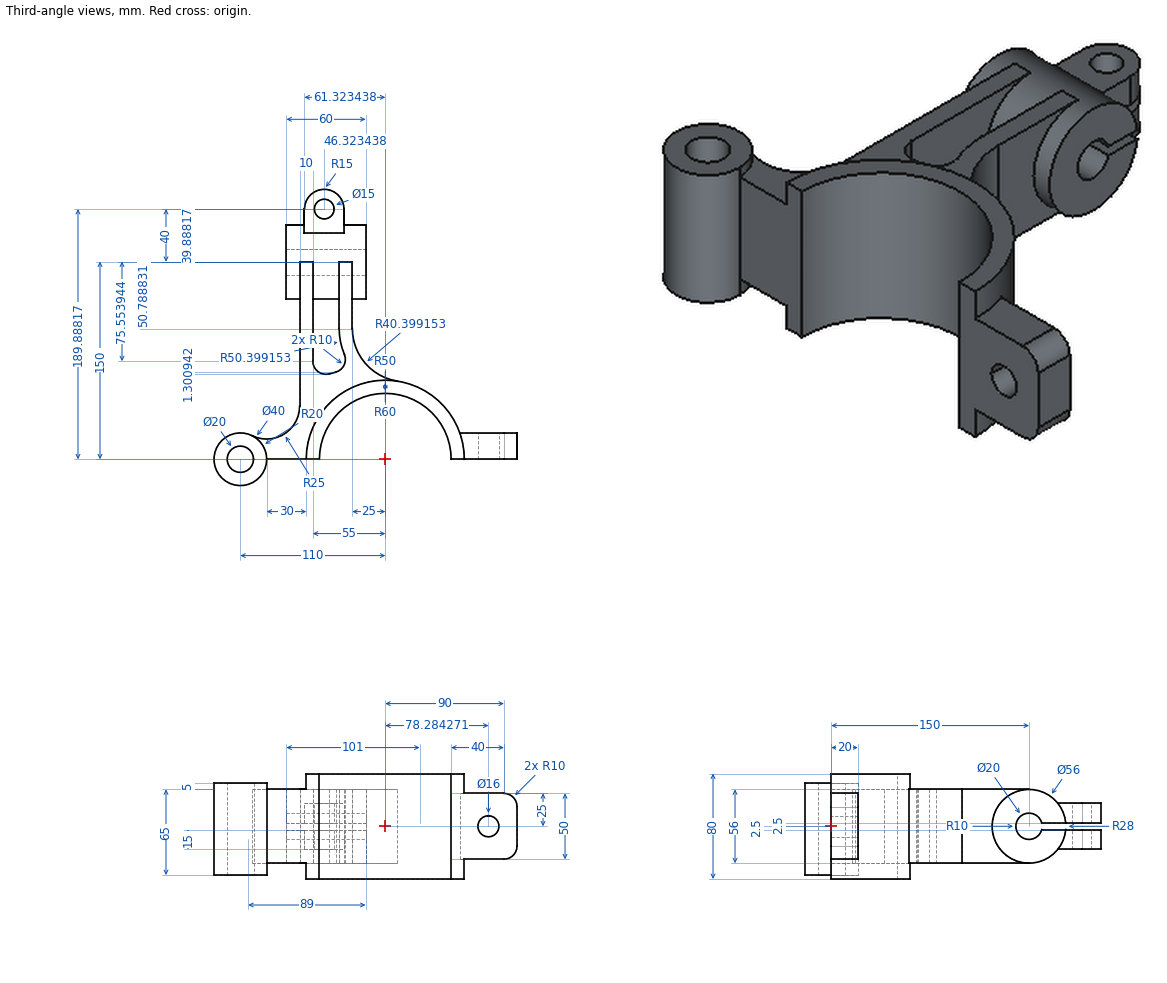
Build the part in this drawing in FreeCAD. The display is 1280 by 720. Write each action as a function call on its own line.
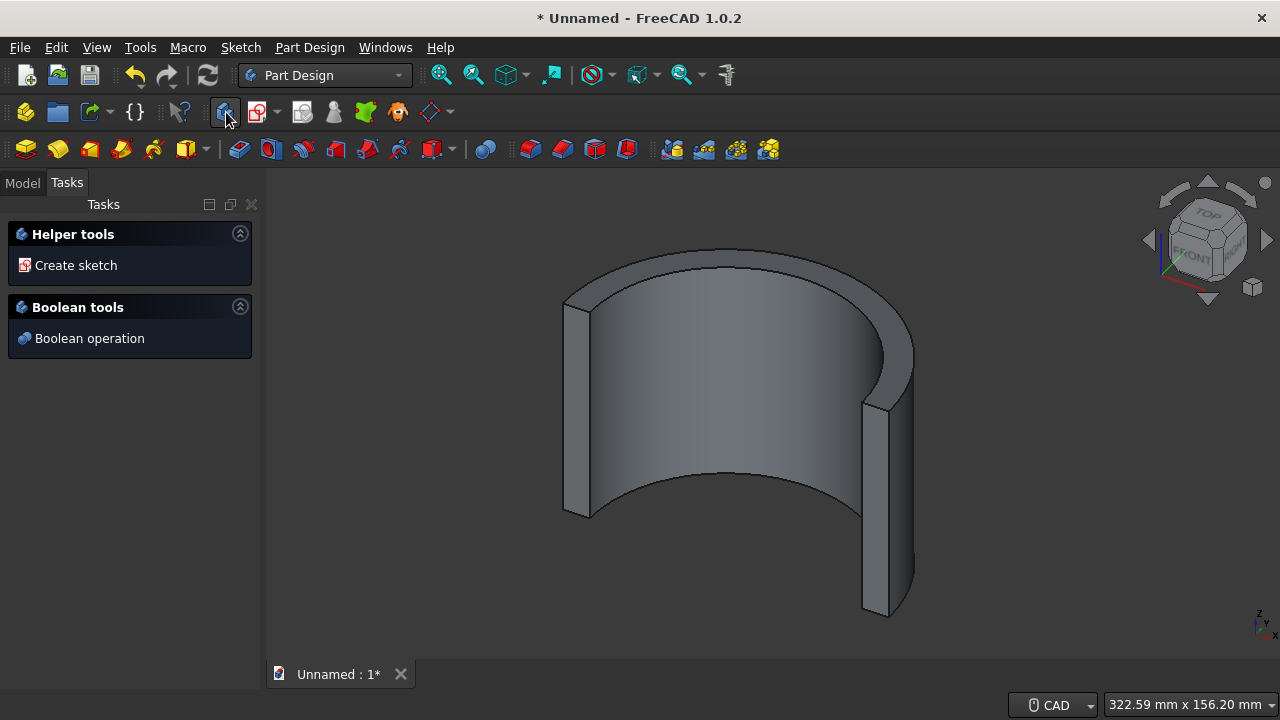
click(23, 182)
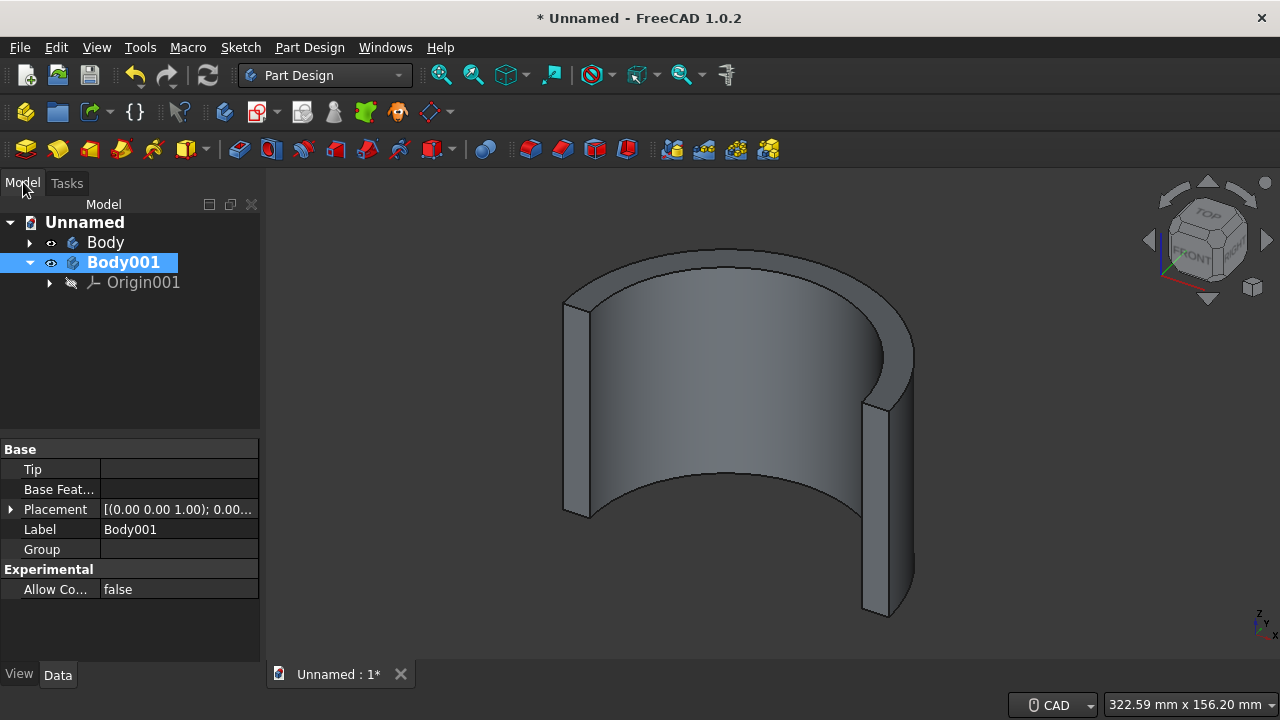
click(50, 283)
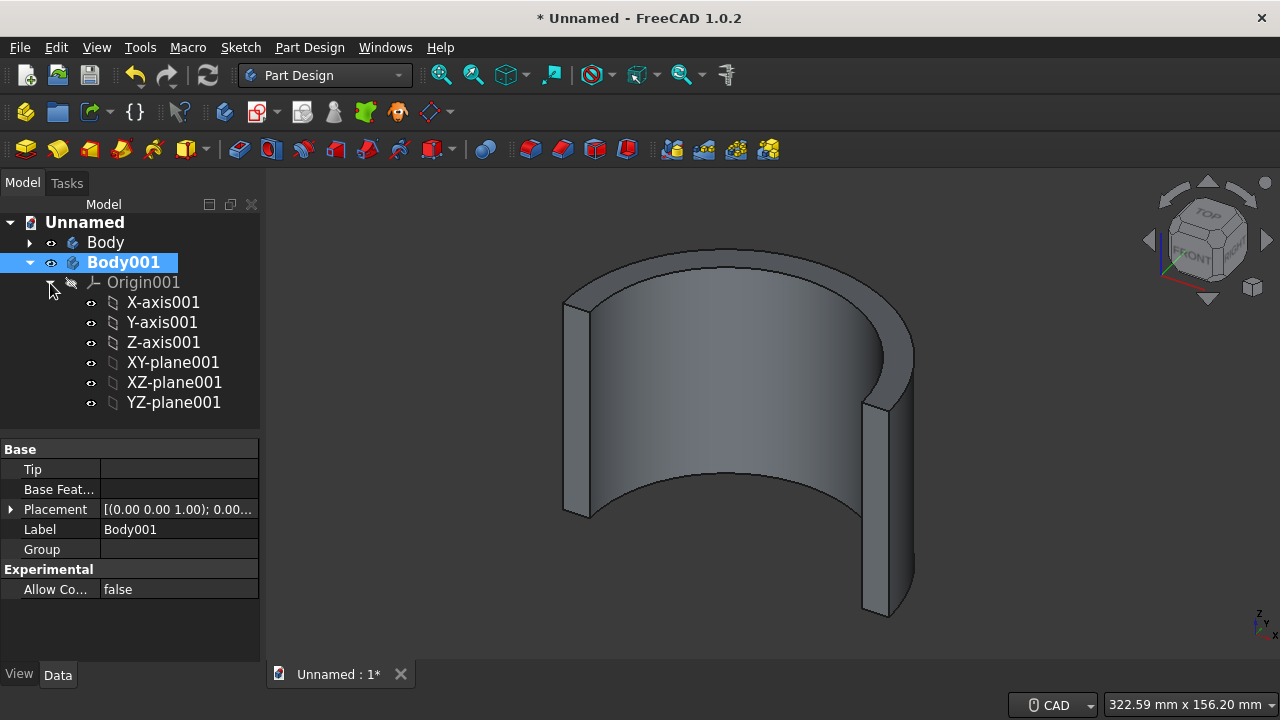
click(136, 363)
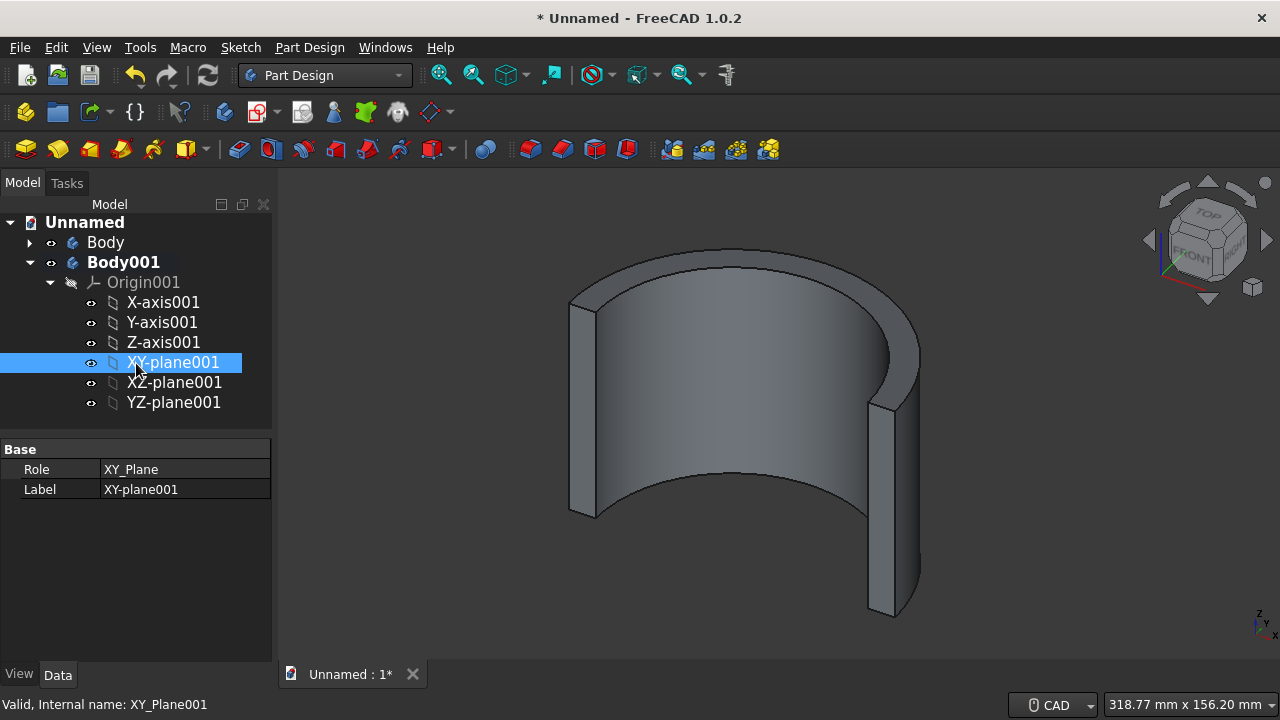
click(430, 112)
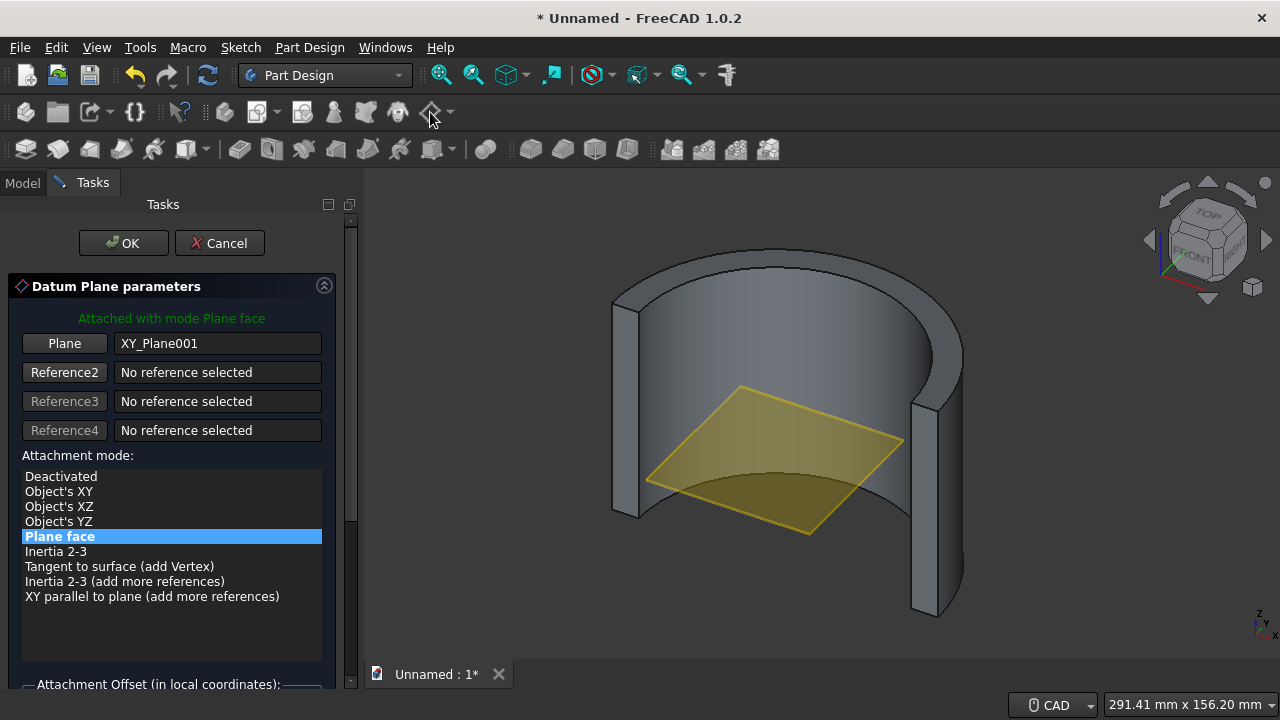
scroll(351, 451, down, 3)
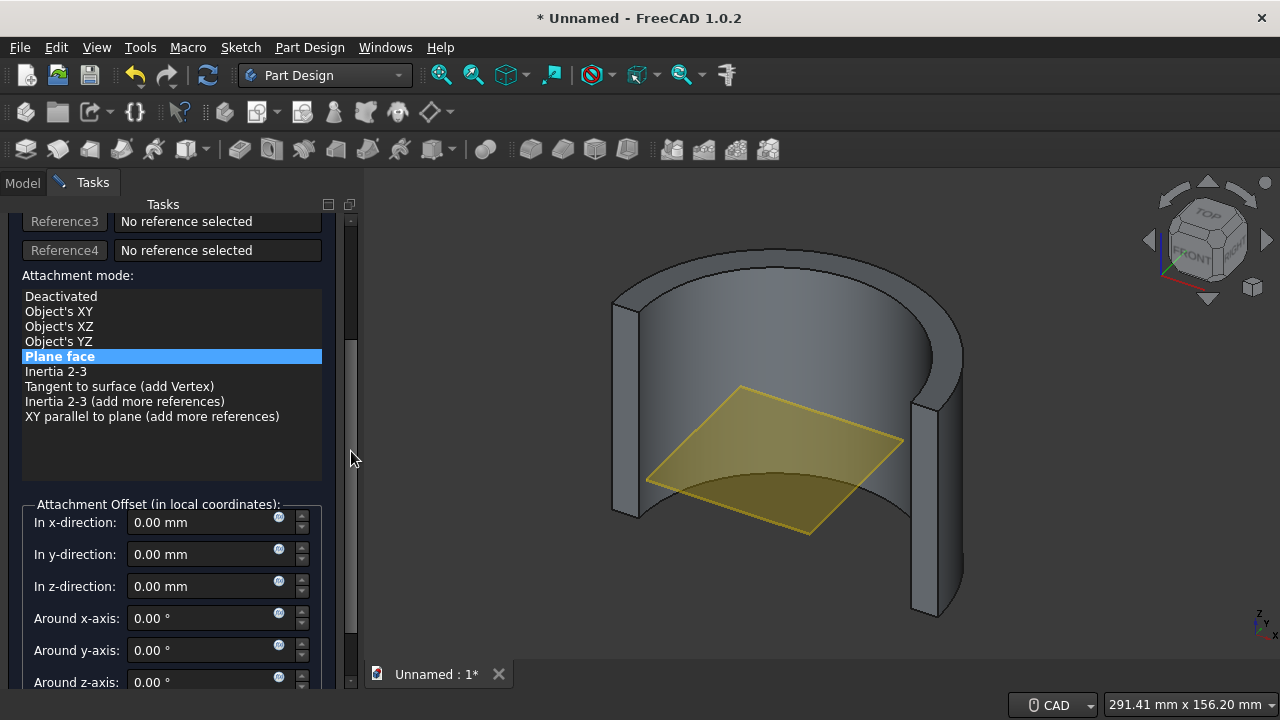
triple_click(210, 586)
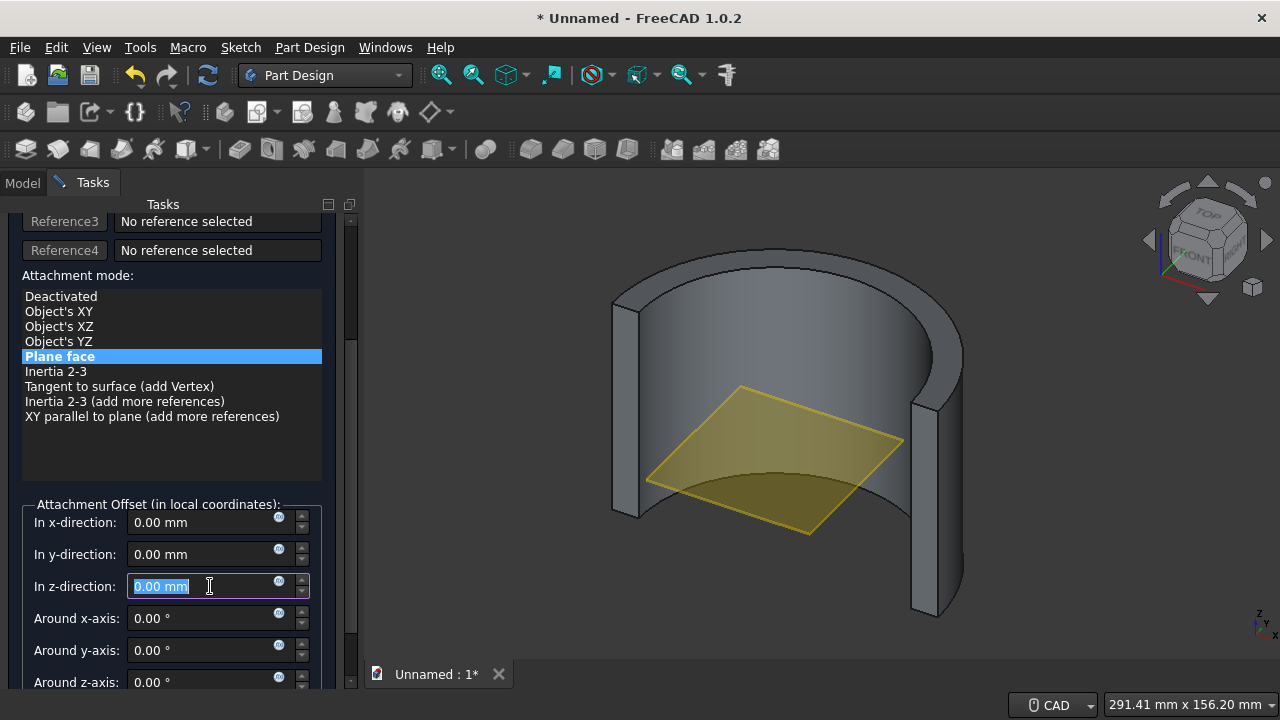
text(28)
key(Tab)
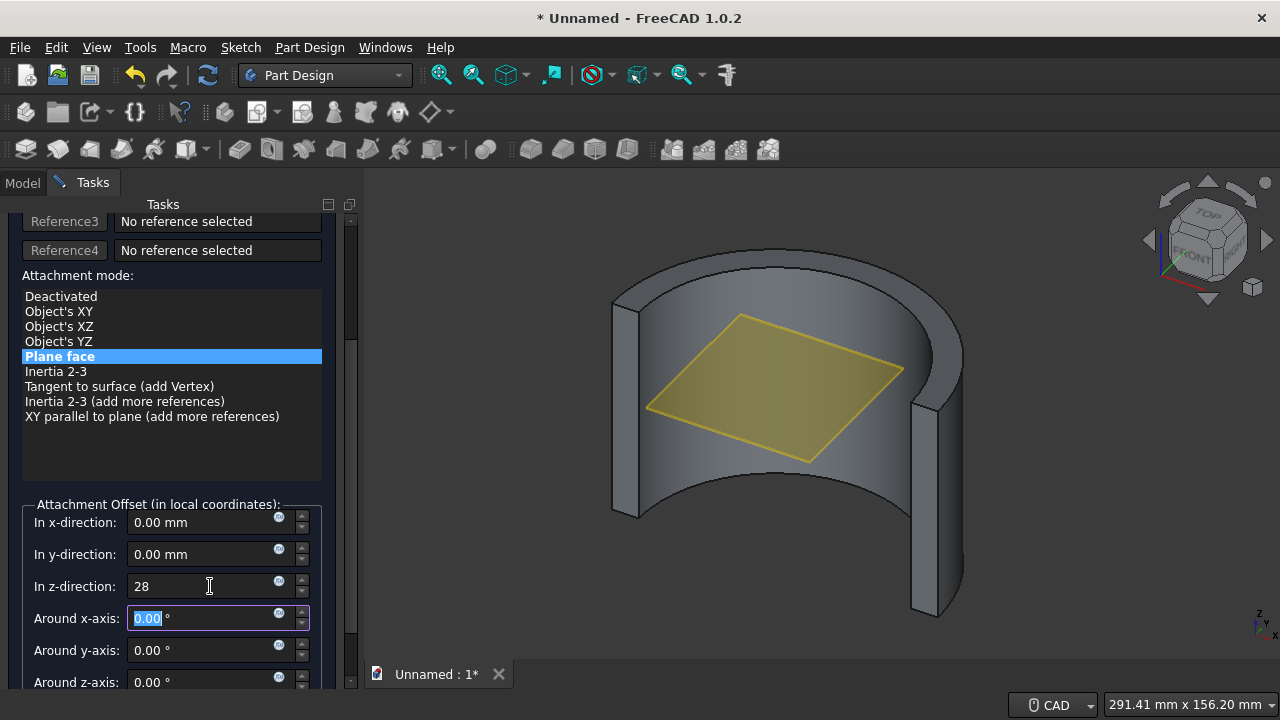
scroll(351, 451, up, 4)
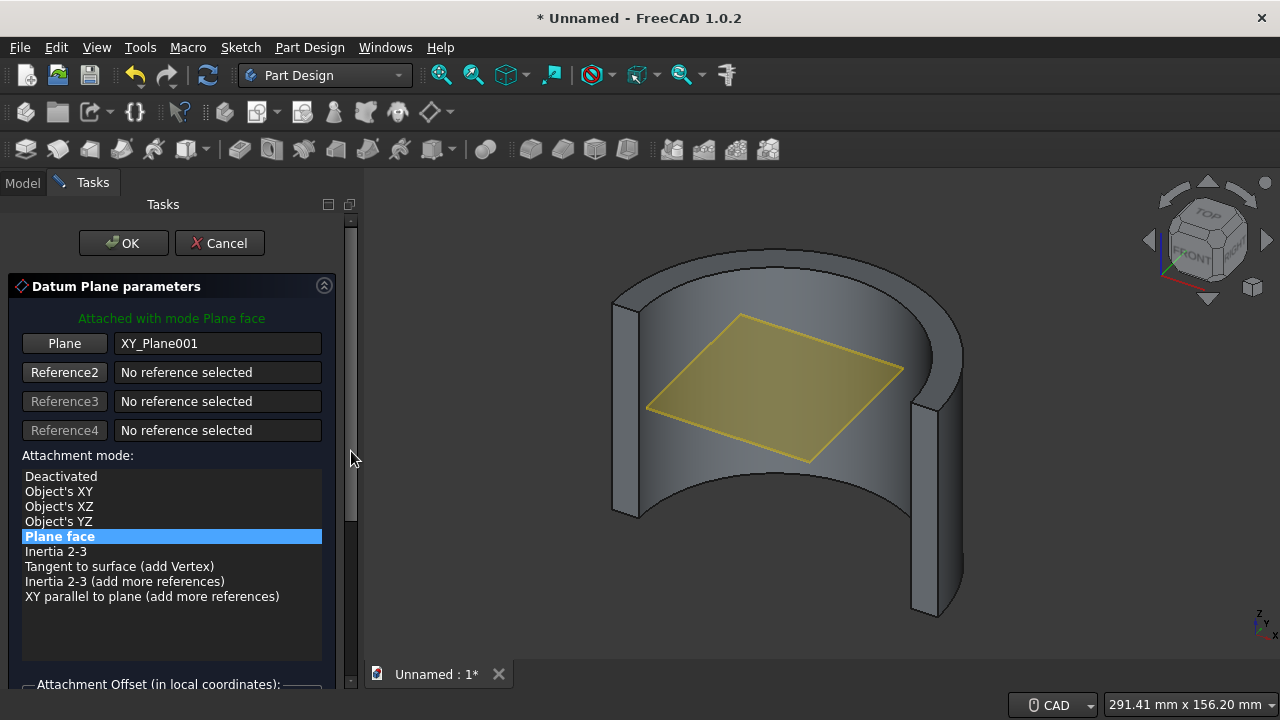
click(124, 243)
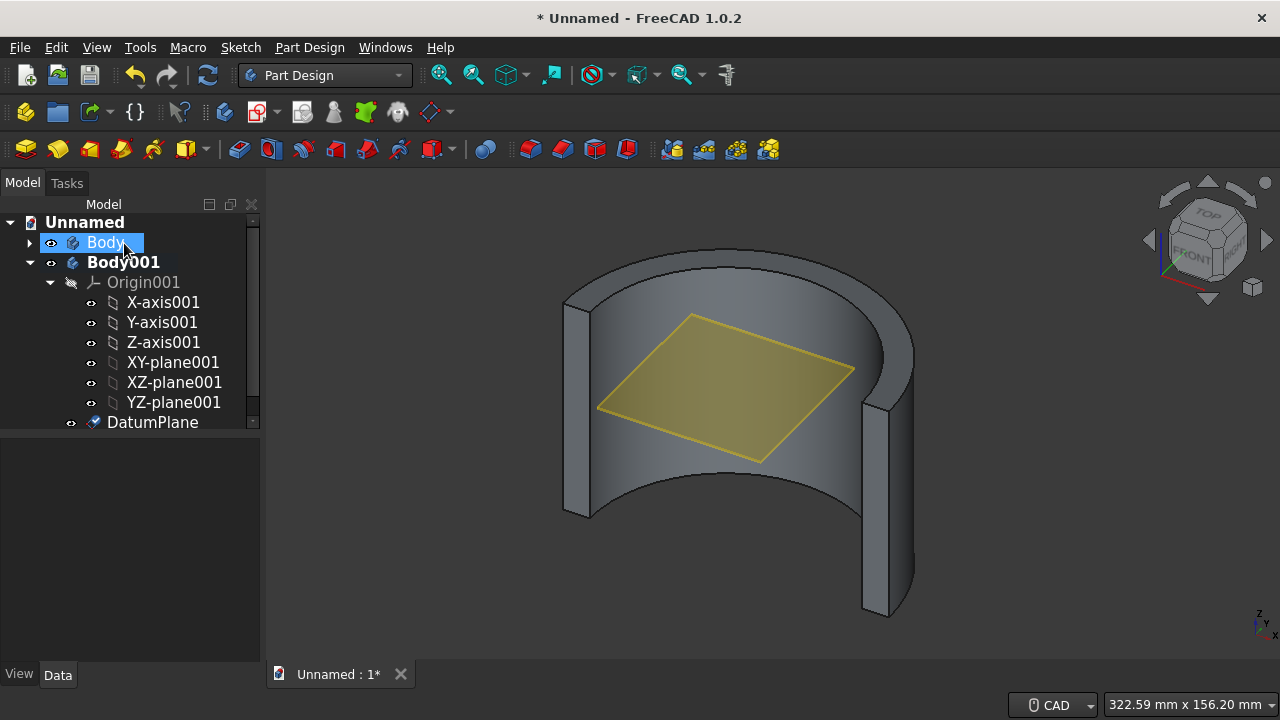
click(116, 423)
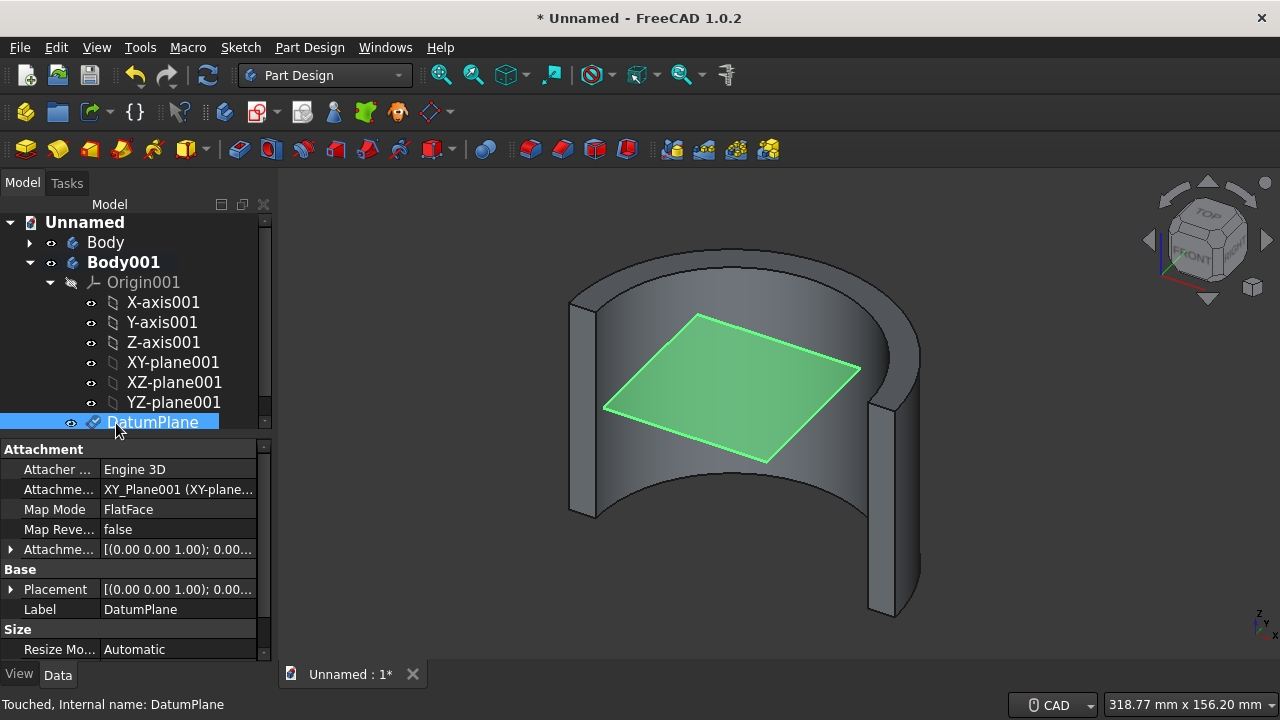
click(258, 112)